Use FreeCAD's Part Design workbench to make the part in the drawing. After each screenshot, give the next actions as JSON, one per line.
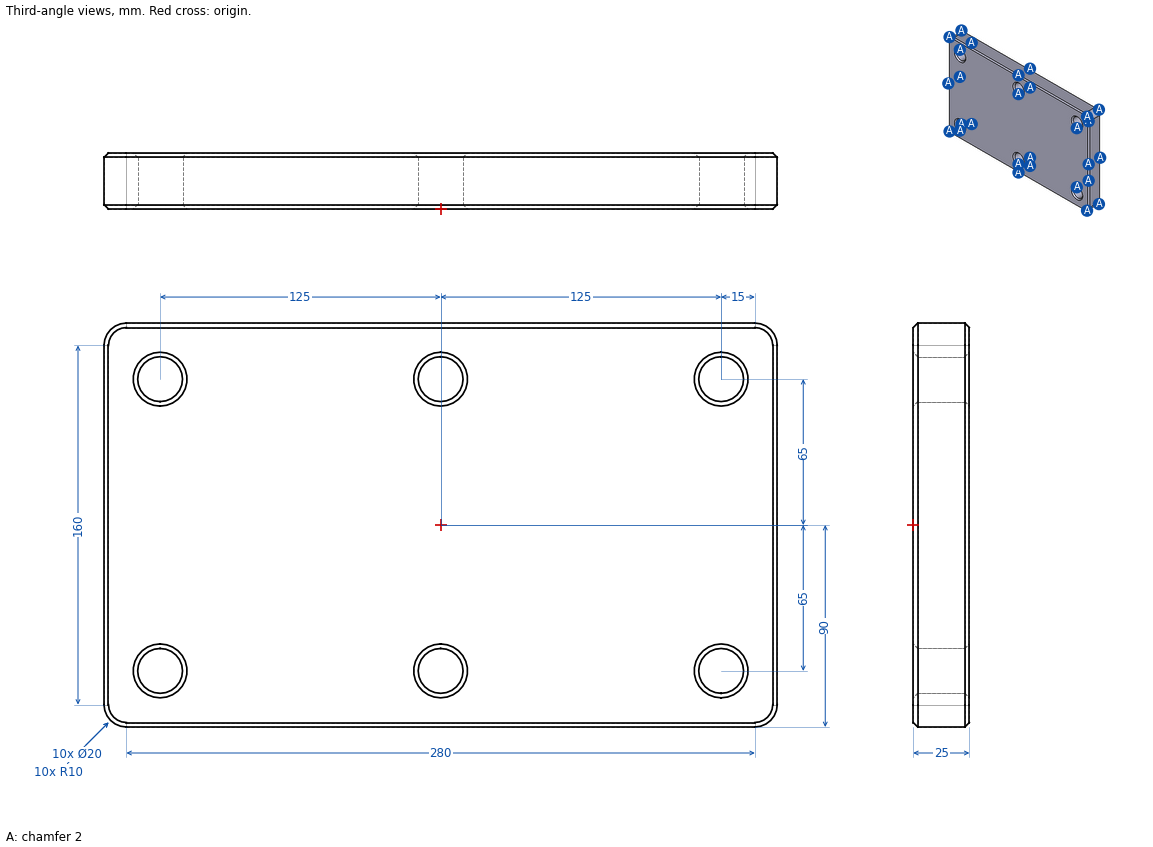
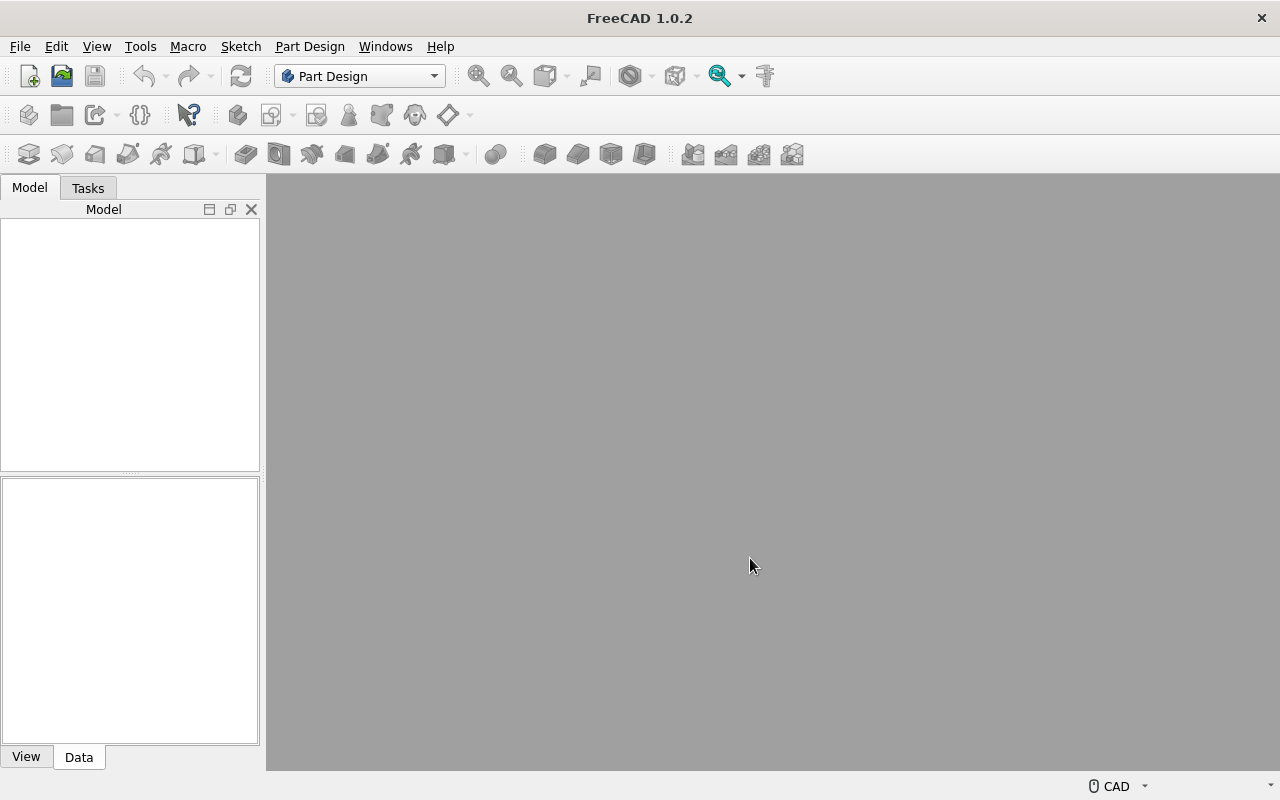
{"action": "left_click", "coordinate": [29, 76]}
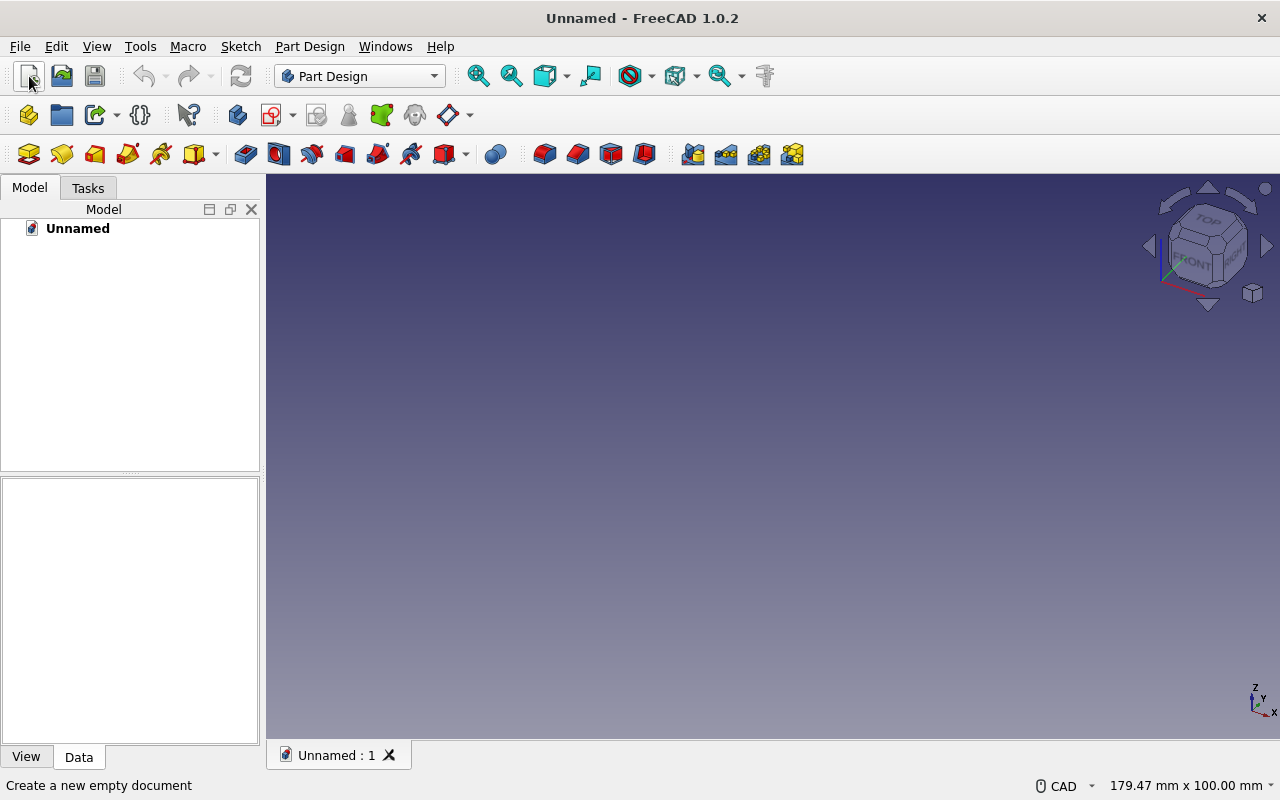
{"action": "left_click", "coordinate": [270, 116]}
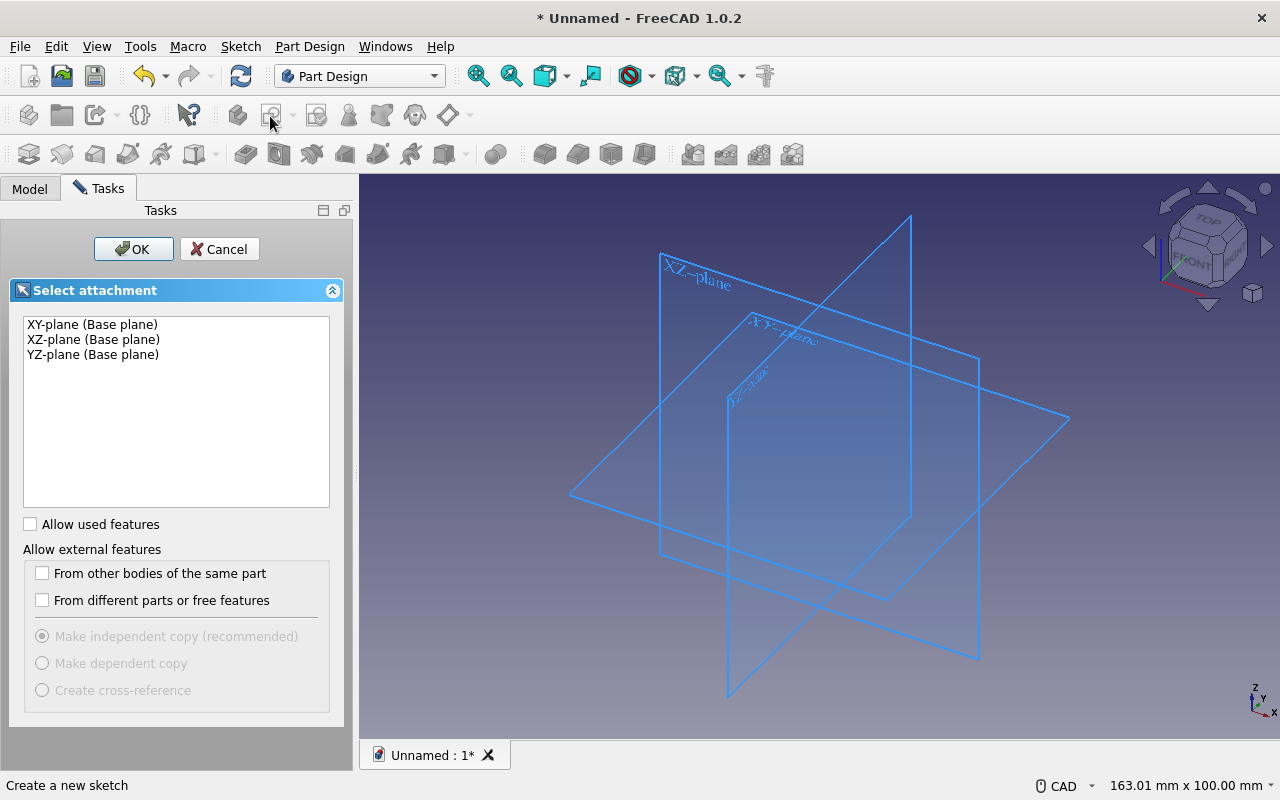
{"action": "left_click", "coordinate": [84, 340]}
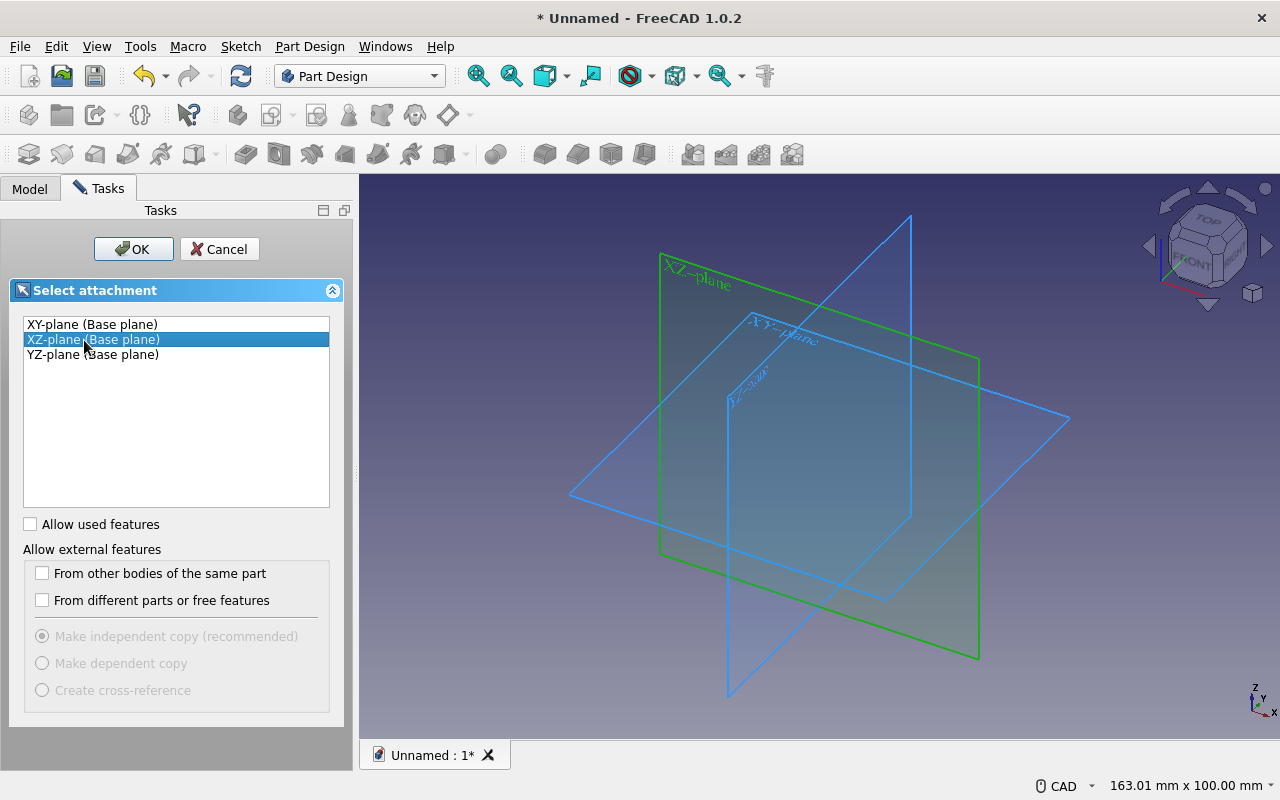
{"action": "left_click", "coordinate": [134, 249]}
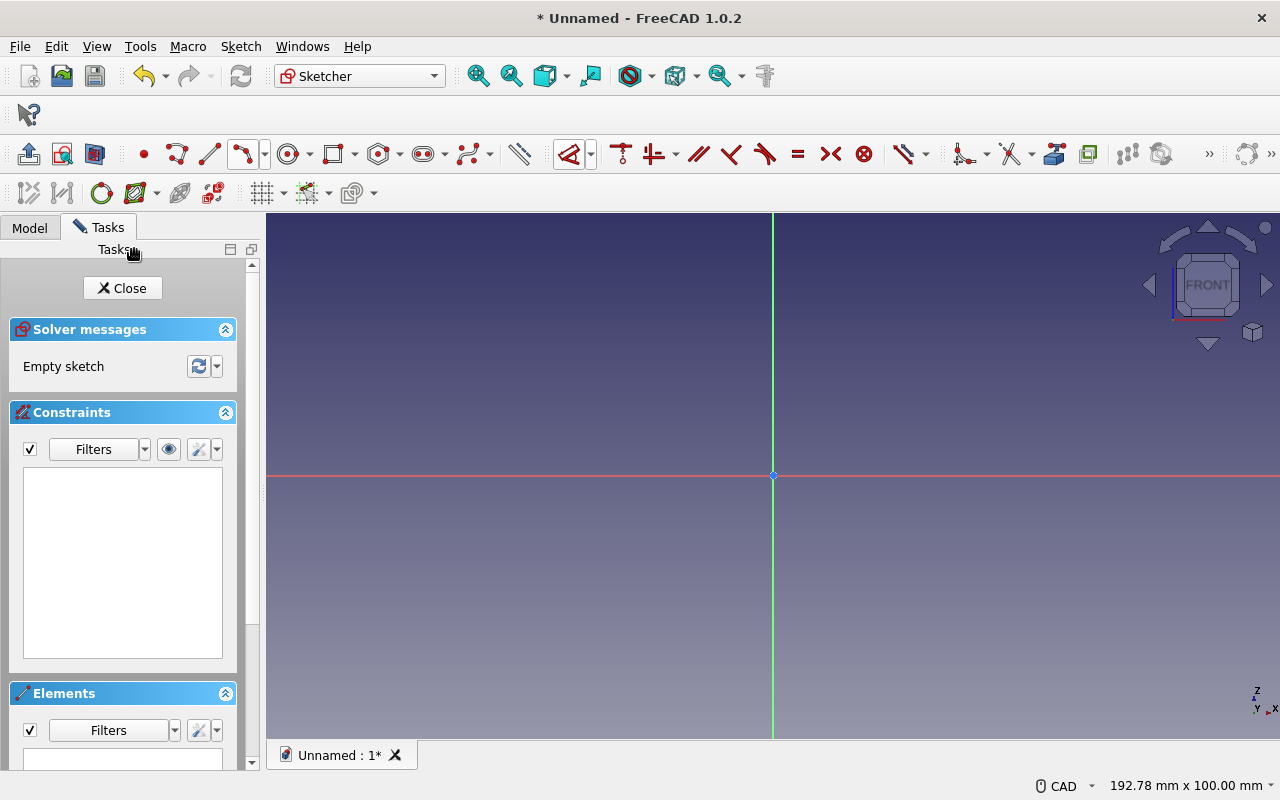
{"action": "scroll", "coordinate": [665, 476], "scroll_direction": "down", "scroll_amount": 5}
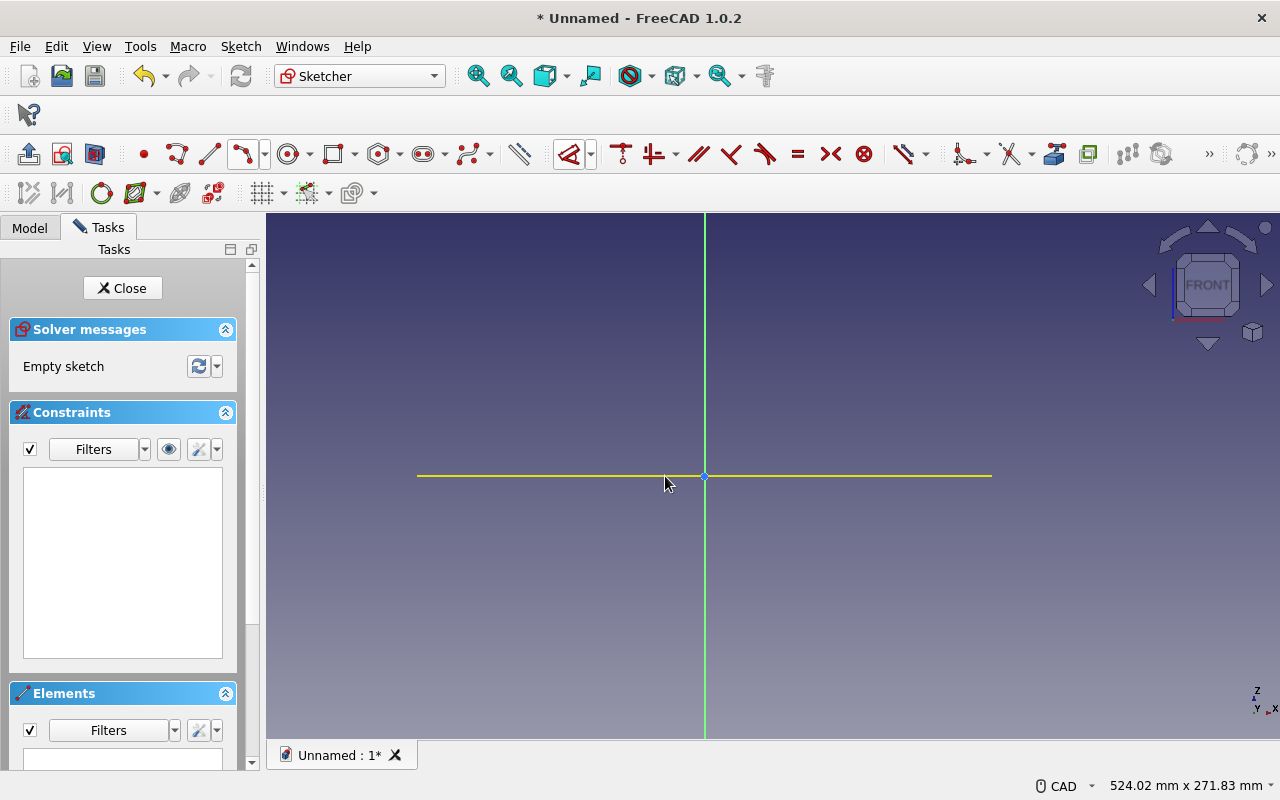
{"action": "left_click", "coordinate": [210, 154]}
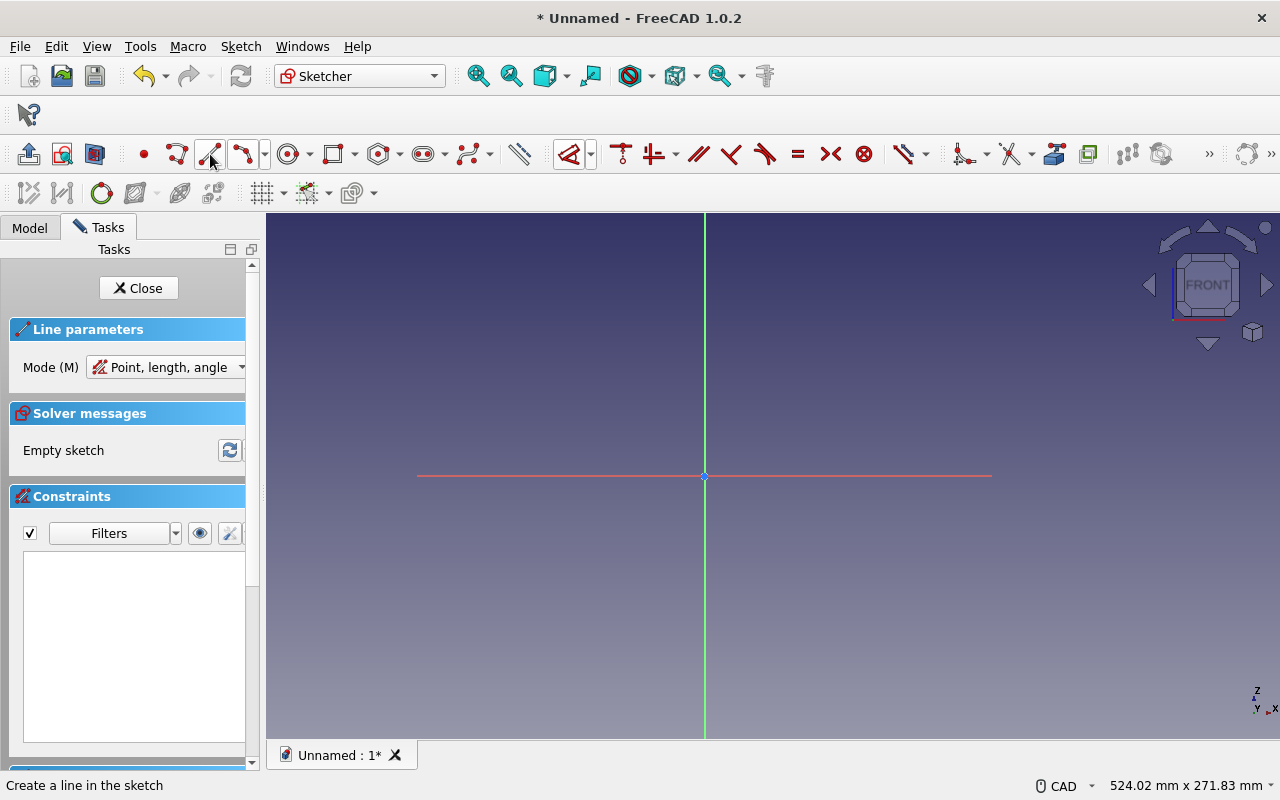
{"action": "left_click", "coordinate": [976, 650]}
{"action": "left_click", "coordinate": [434, 650]}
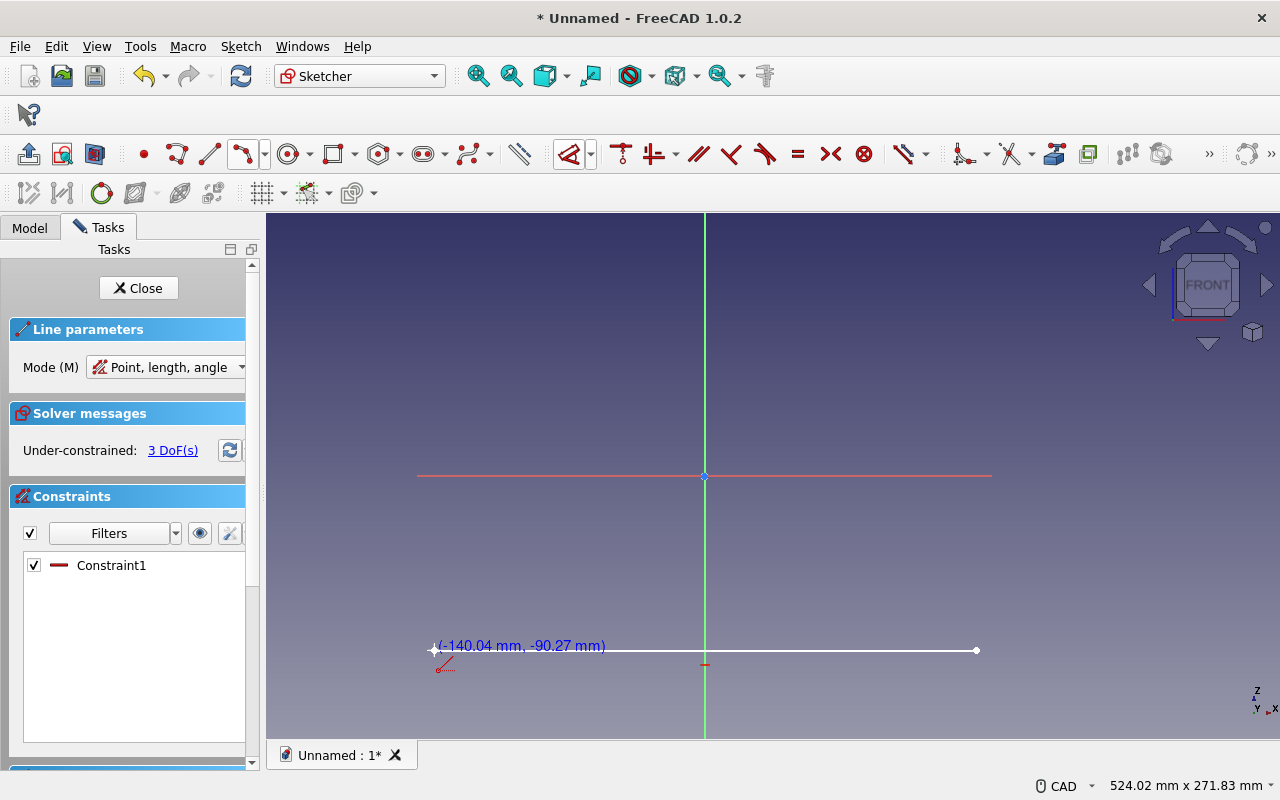
{"action": "left_click", "coordinate": [415, 631]}
{"action": "left_click", "coordinate": [415, 322]}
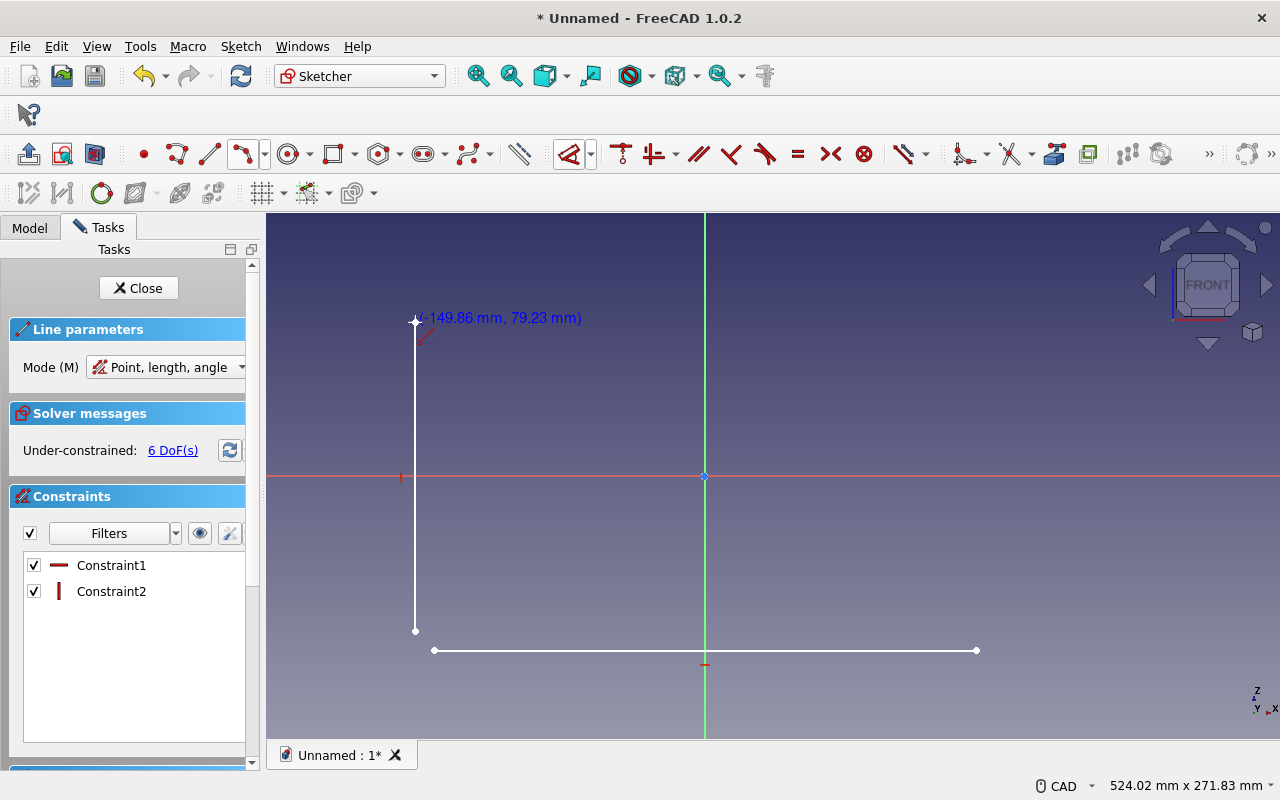
{"action": "left_click", "coordinate": [434, 302]}
{"action": "left_click", "coordinate": [976, 302]}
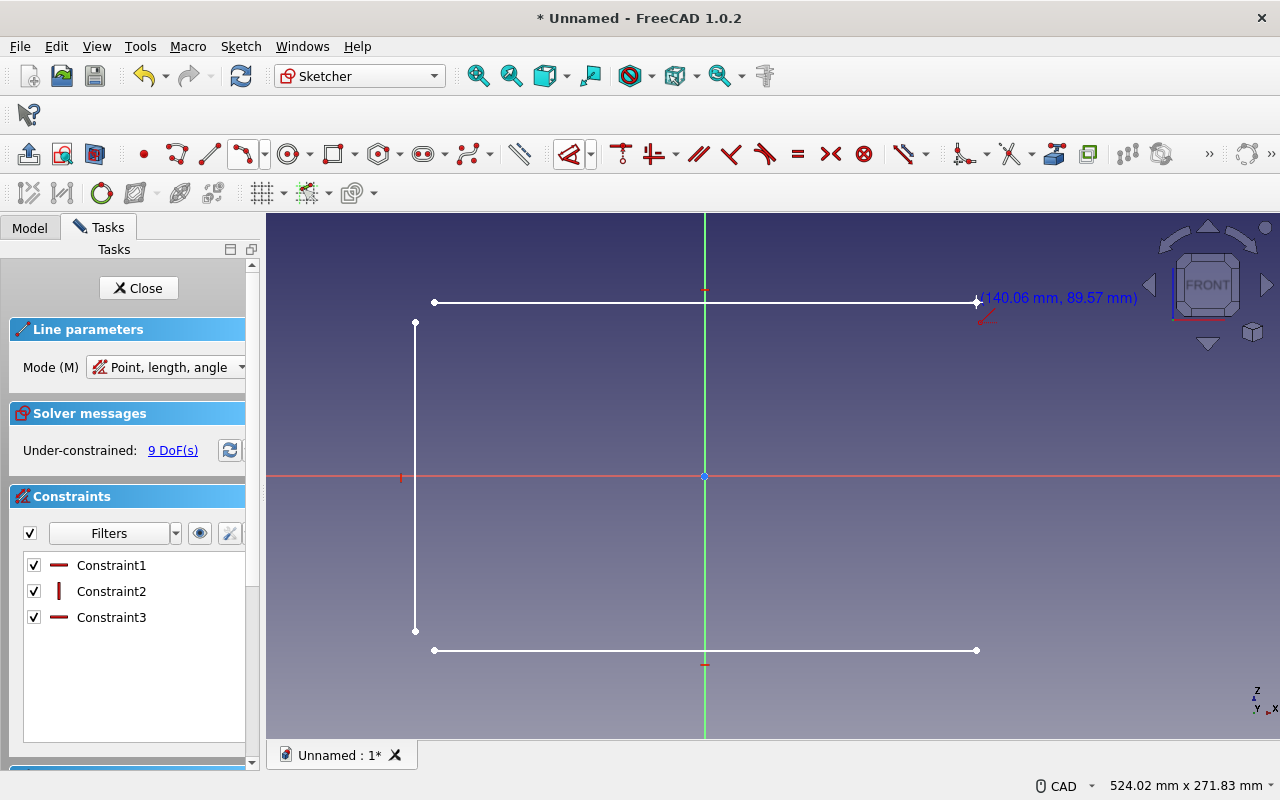
{"action": "left_click", "coordinate": [995, 322]}
{"action": "left_click", "coordinate": [995, 631]}